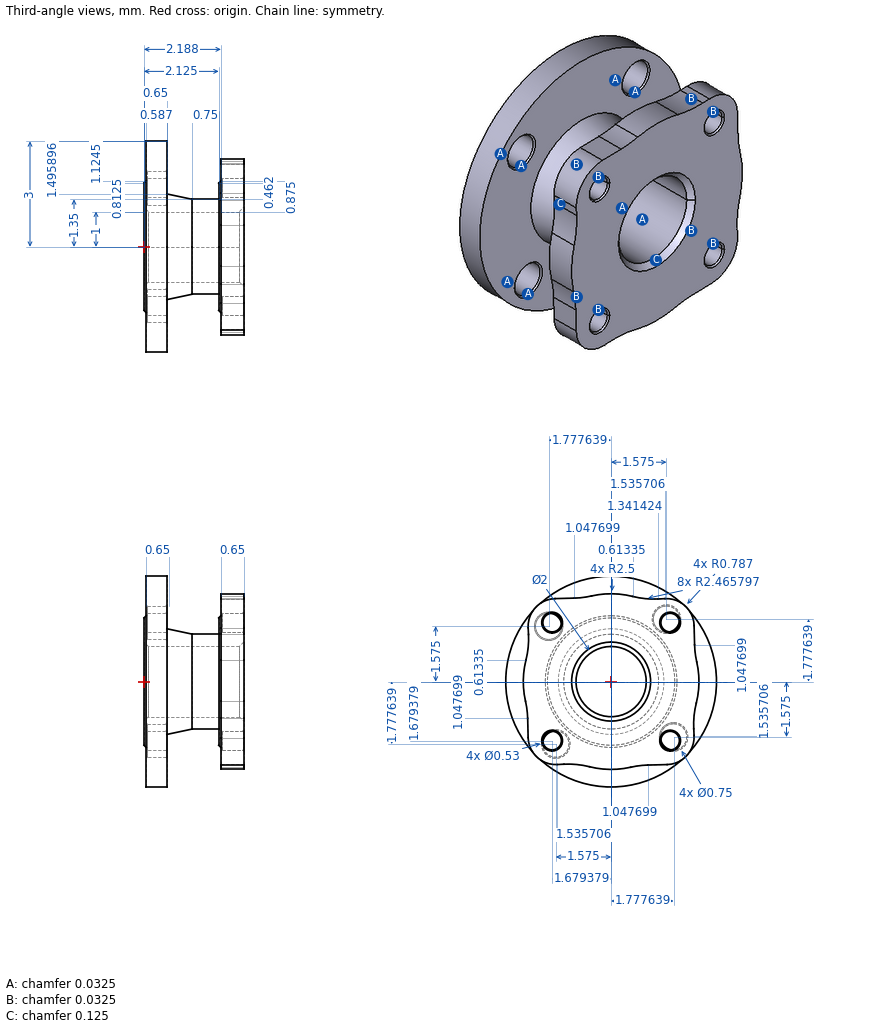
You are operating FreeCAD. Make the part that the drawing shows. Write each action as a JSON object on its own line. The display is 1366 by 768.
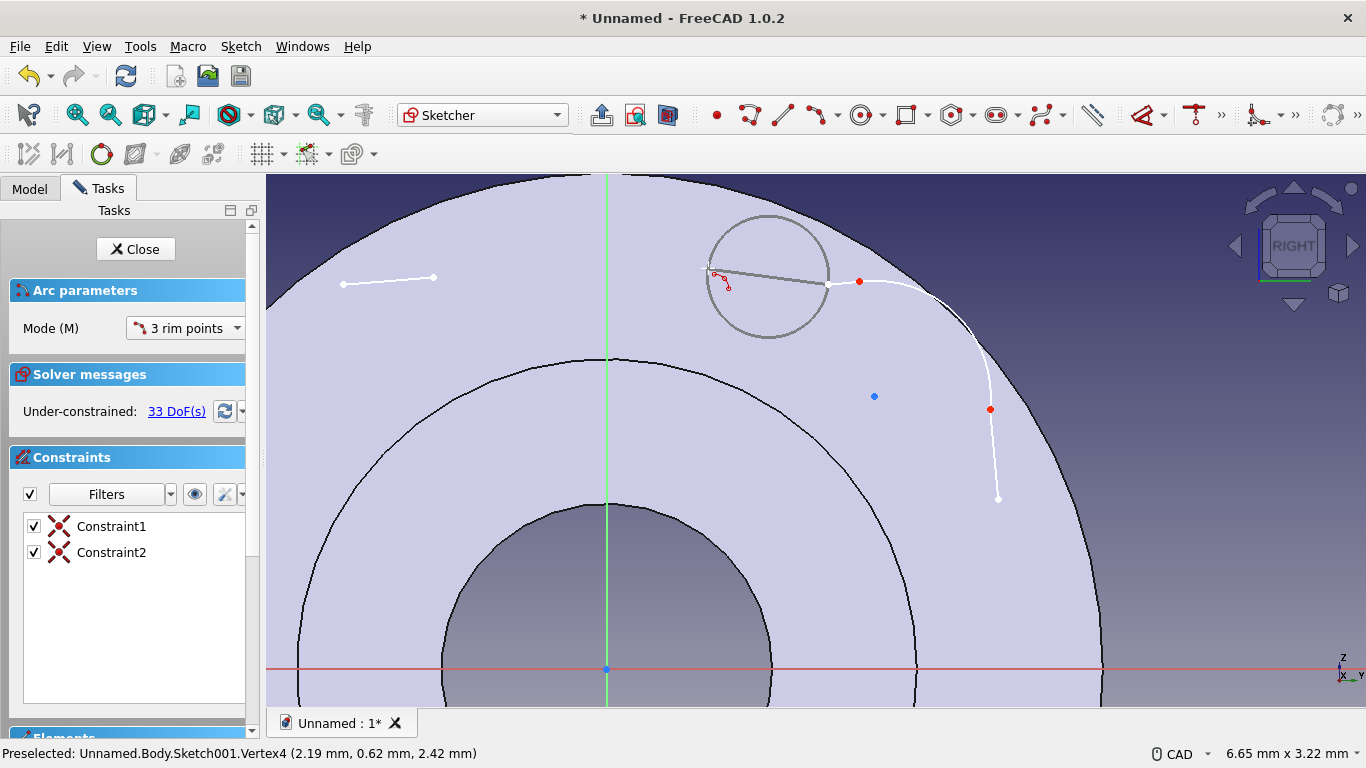
{"action": "scroll", "coordinate": [768, 279], "scroll_direction": "up", "scroll_amount": 7}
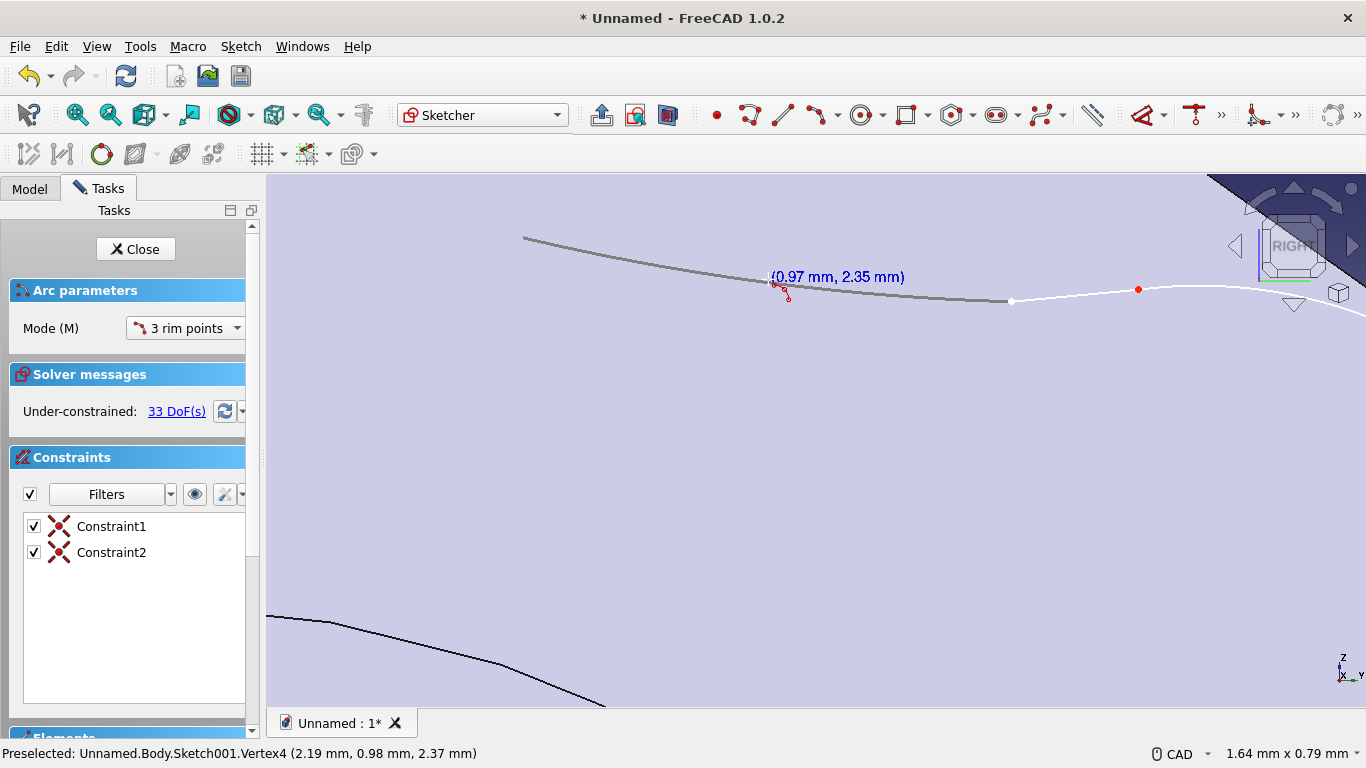
{"action": "left_click", "coordinate": [767, 278]}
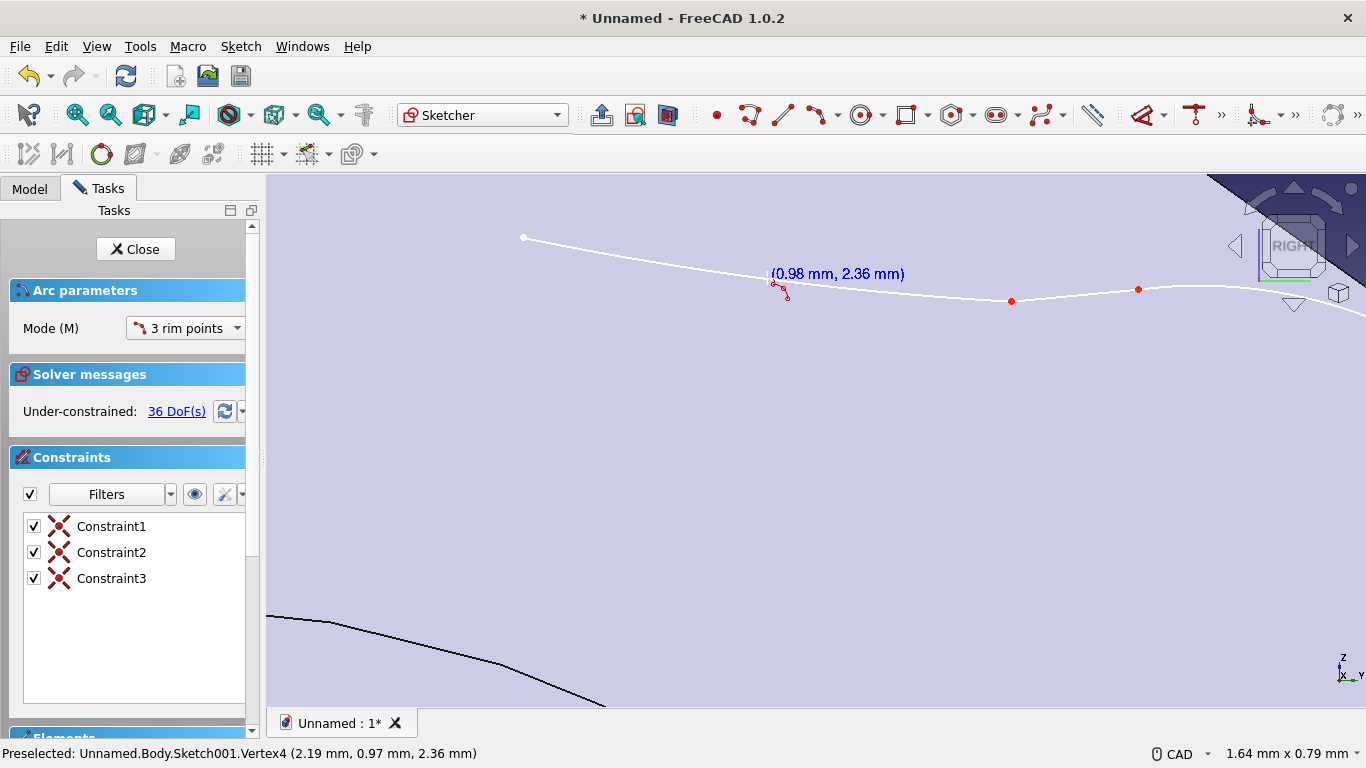
{"action": "scroll", "coordinate": [827, 264], "scroll_direction": "down", "scroll_amount": 11}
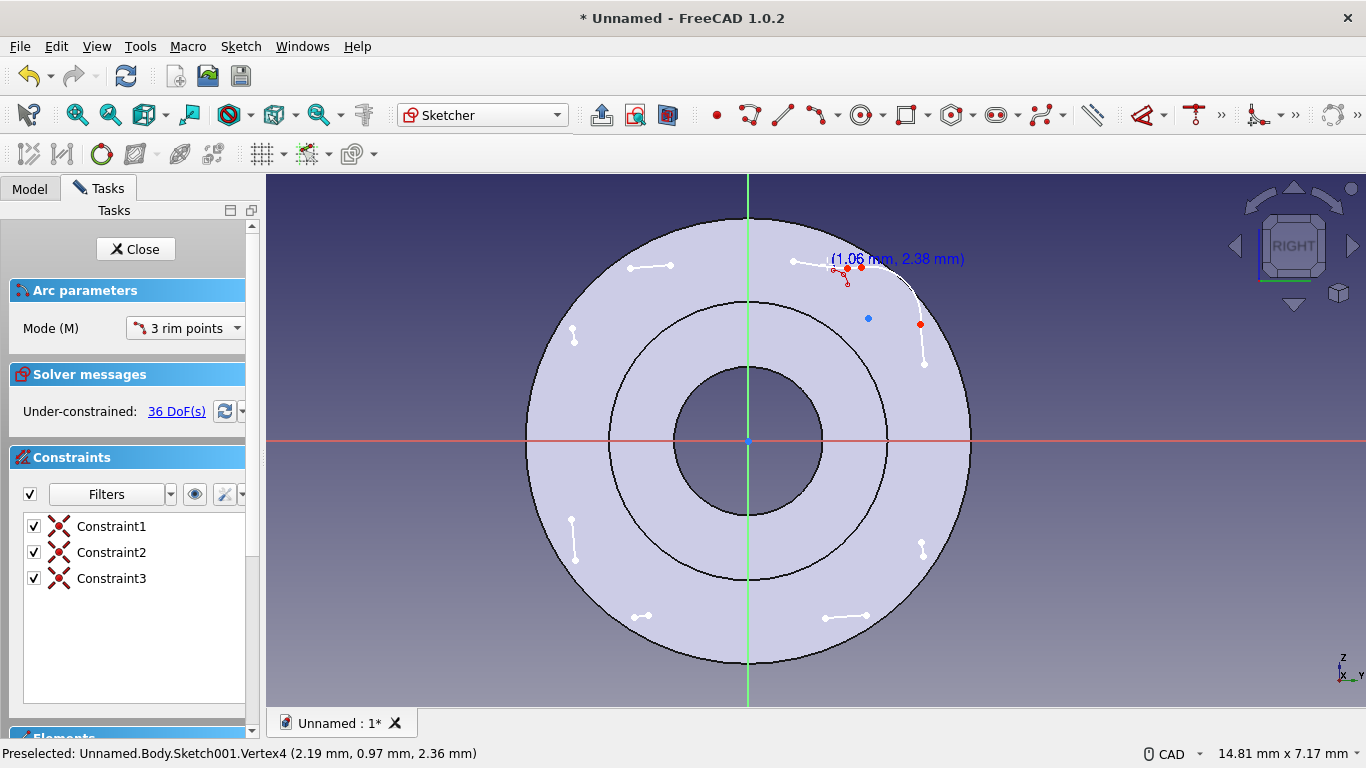
{"action": "left_click", "coordinate": [794, 261]}
{"action": "left_click", "coordinate": [707, 260]}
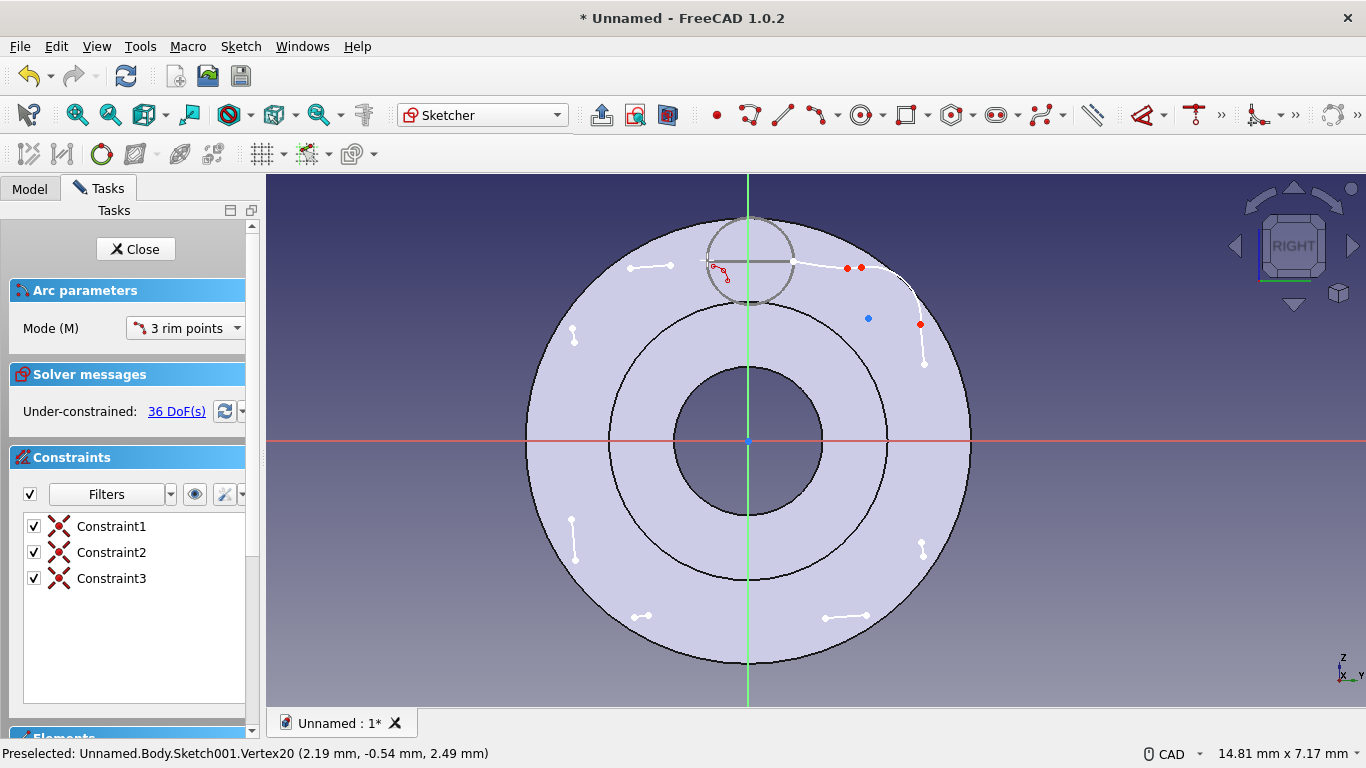
{"action": "scroll", "coordinate": [742, 255], "scroll_direction": "up", "scroll_amount": 6}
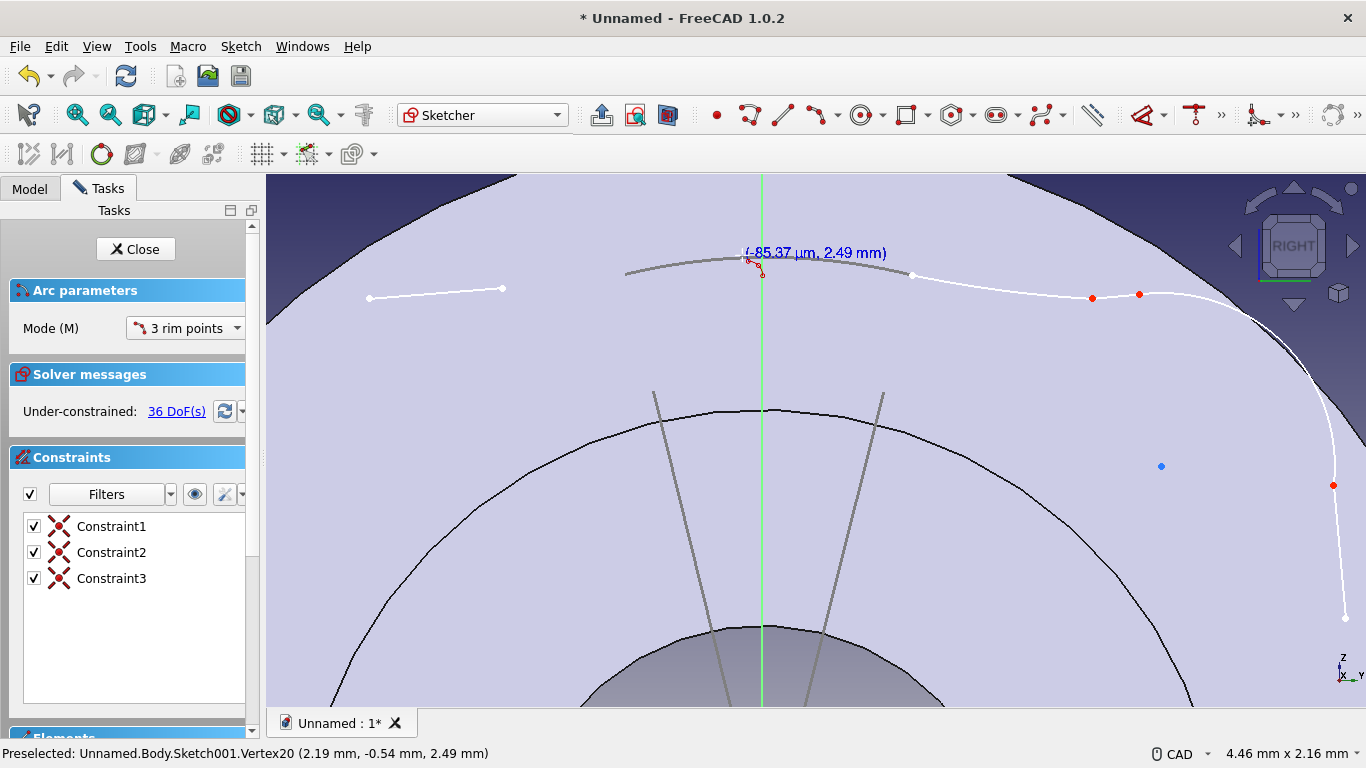
{"action": "left_click", "coordinate": [740, 256]}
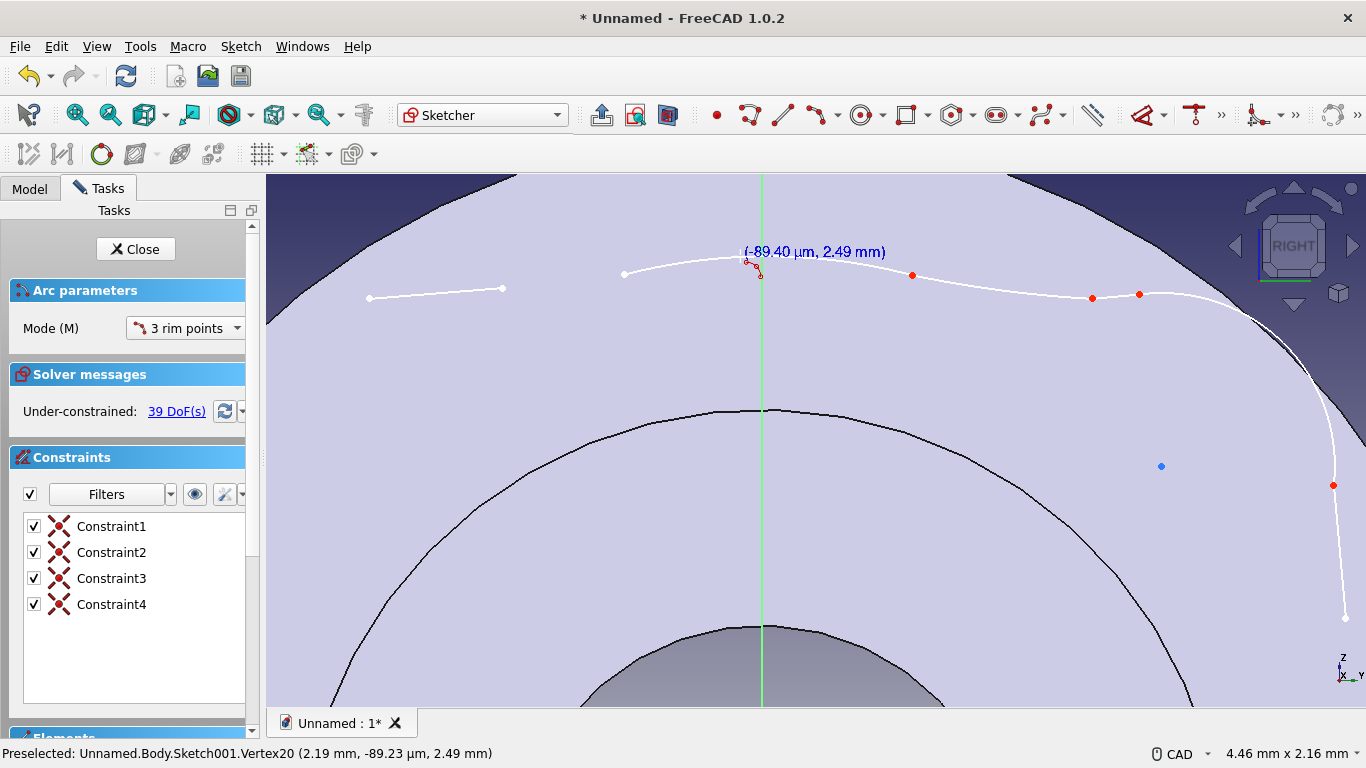
{"action": "scroll", "coordinate": [741, 254], "scroll_direction": "down", "scroll_amount": 6}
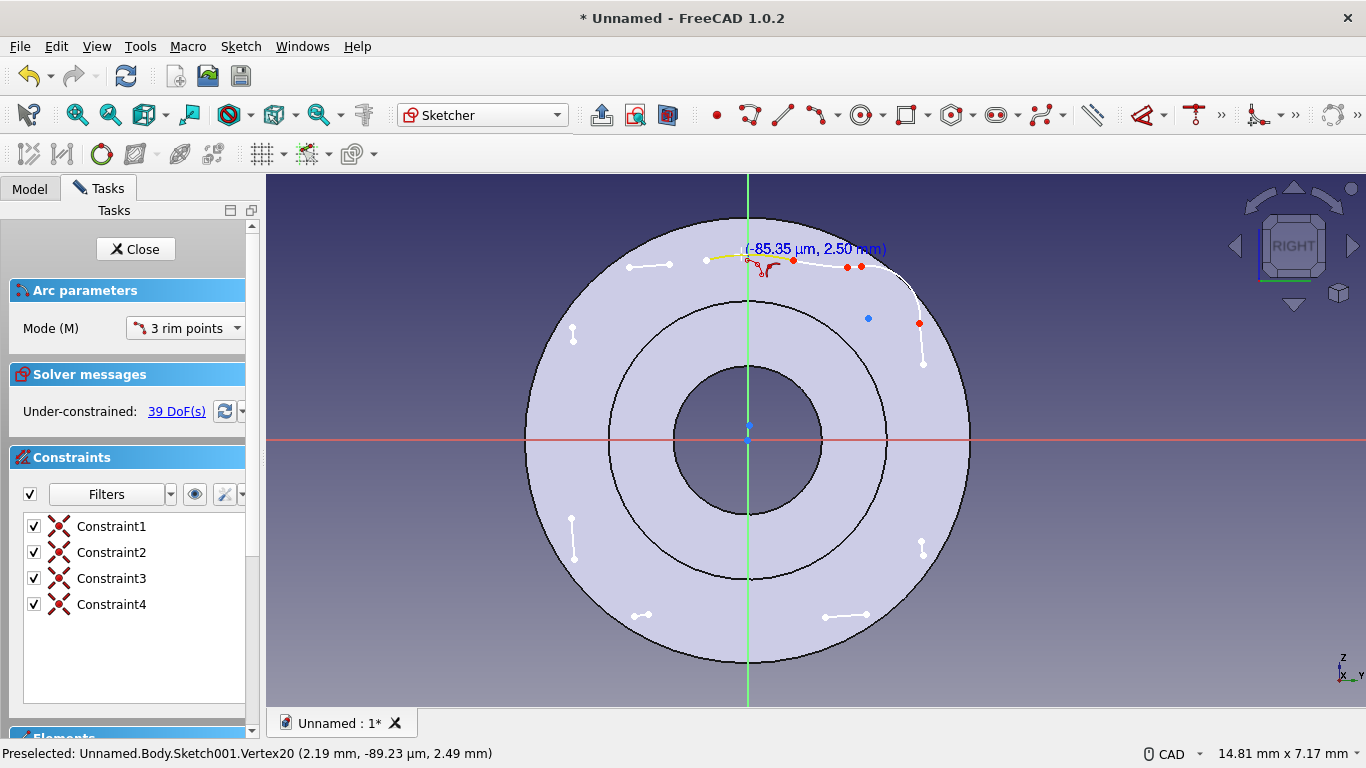
{"action": "left_click", "coordinate": [706, 260]}
{"action": "left_click", "coordinate": [670, 264]}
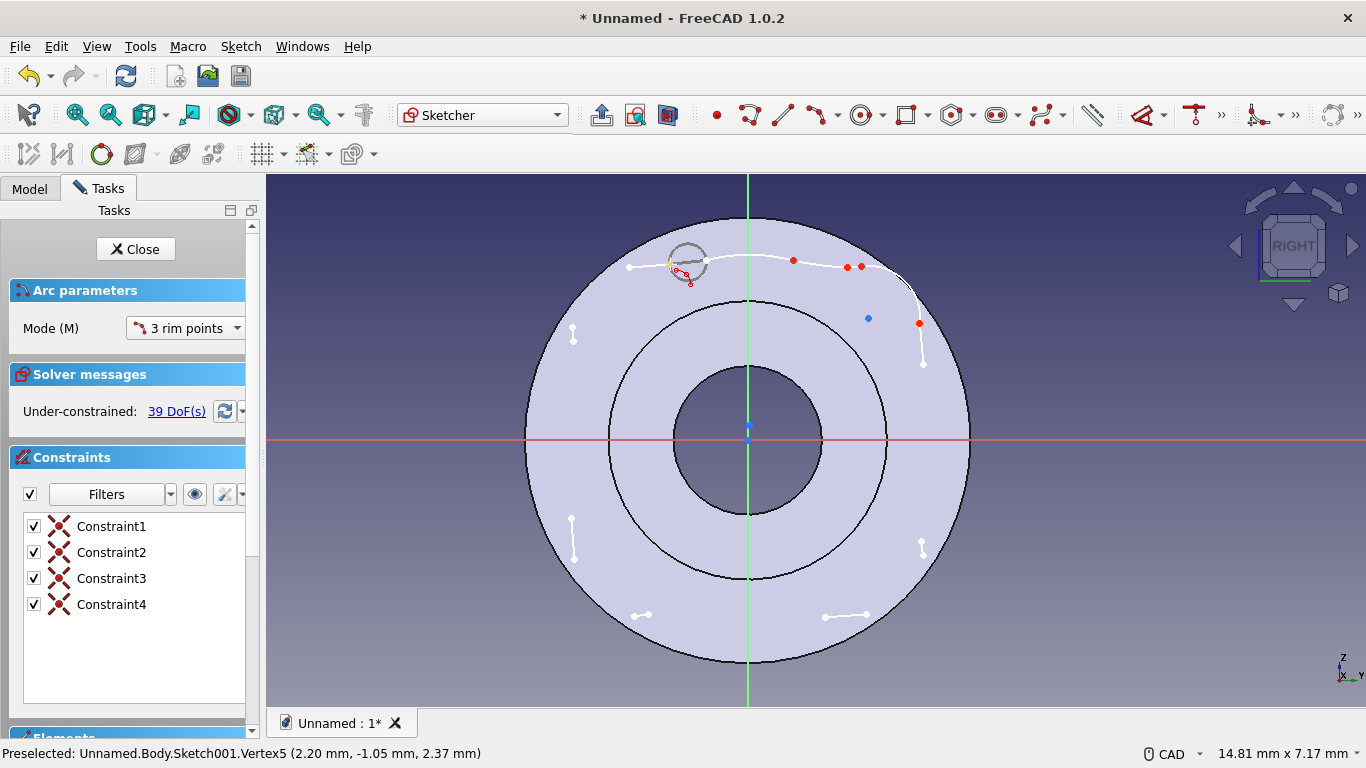
{"action": "scroll", "coordinate": [688, 263], "scroll_direction": "up", "scroll_amount": 15}